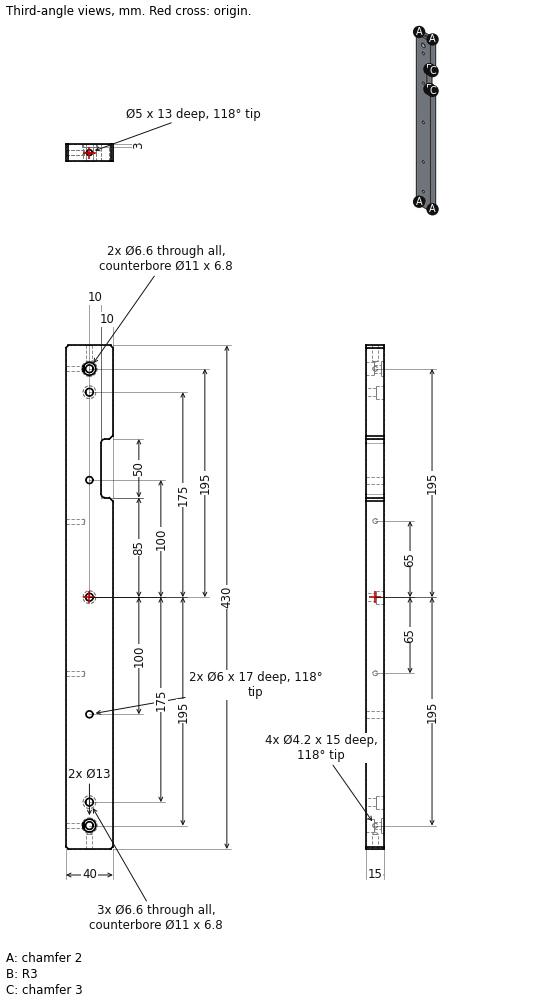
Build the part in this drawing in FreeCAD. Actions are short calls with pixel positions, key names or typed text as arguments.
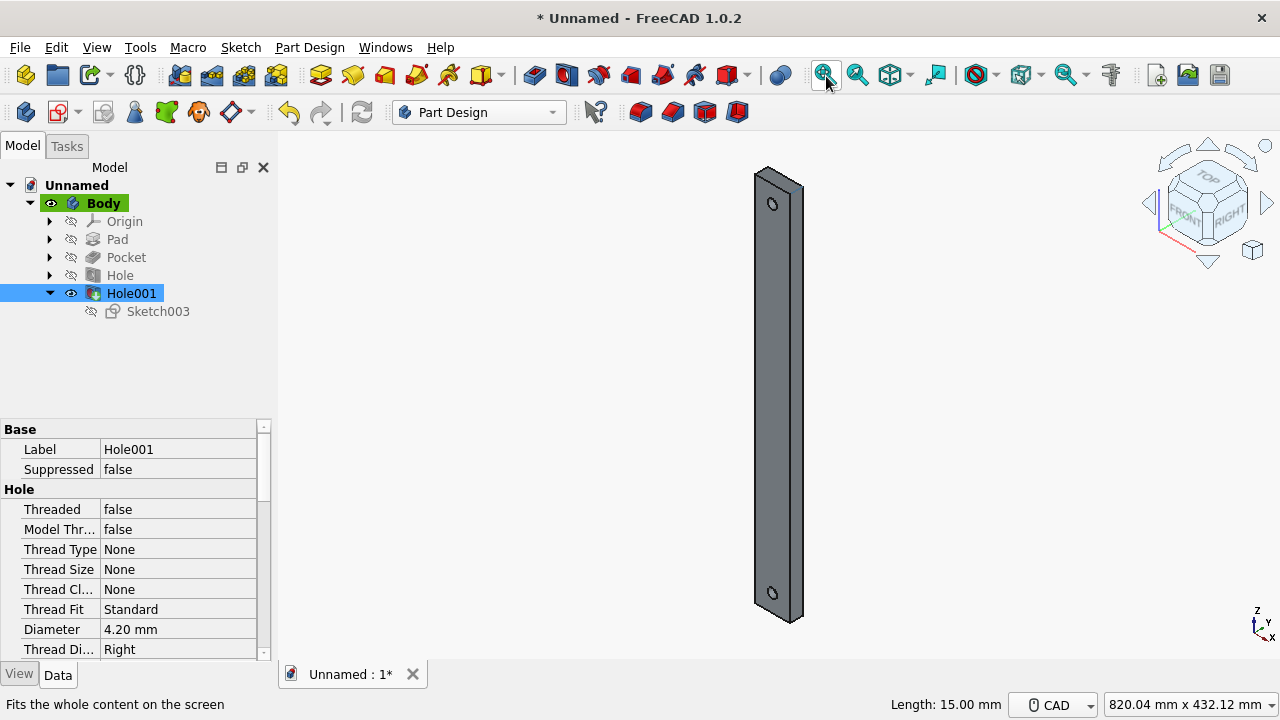
key(2)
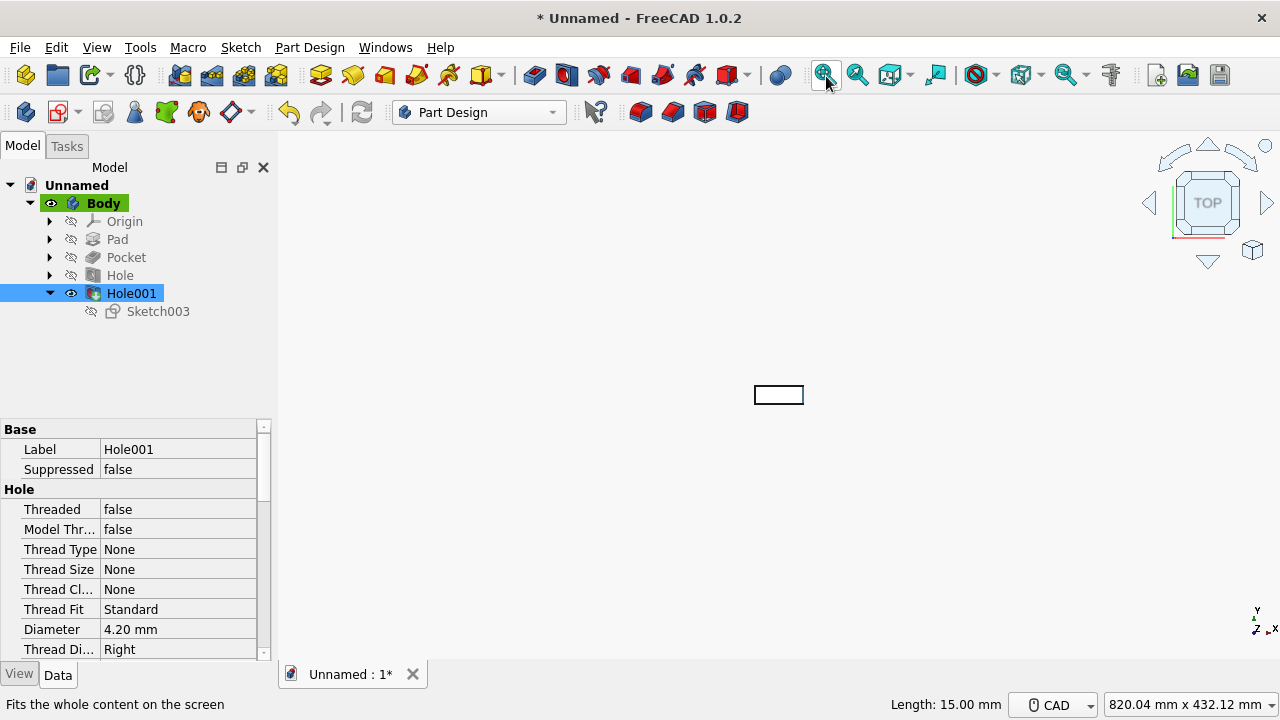
click(826, 76)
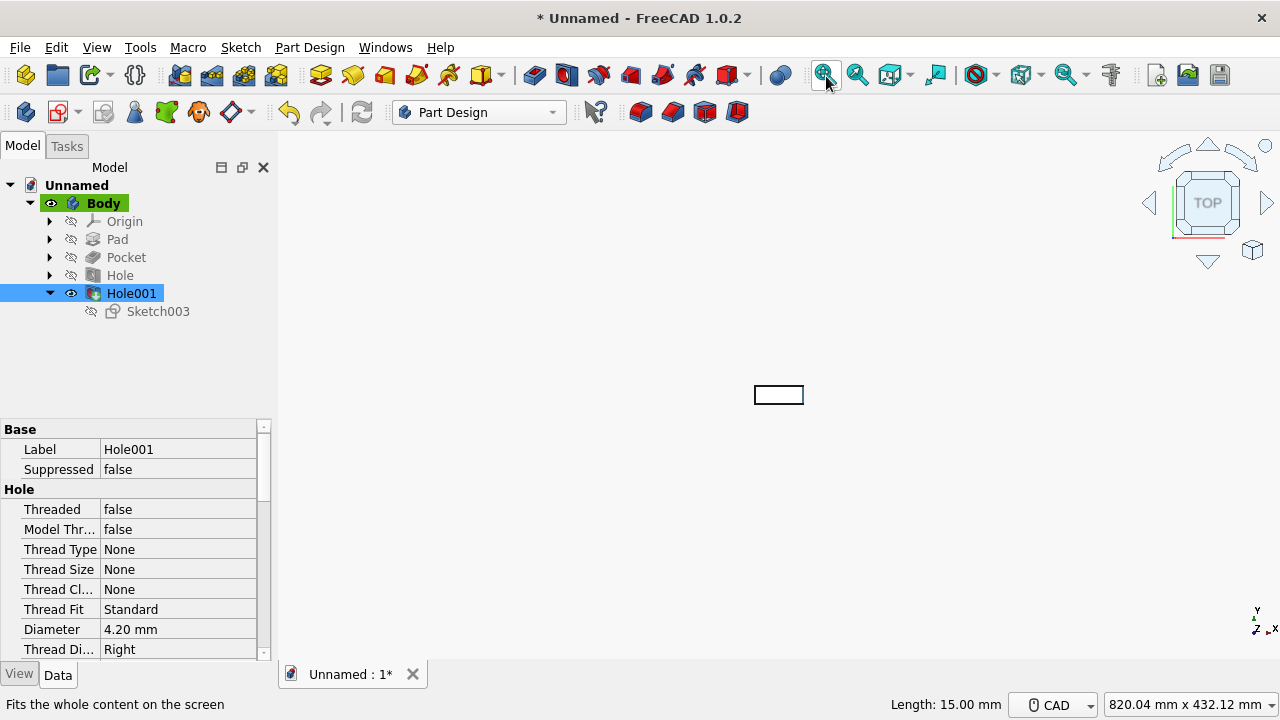
click(755, 394, ctrl)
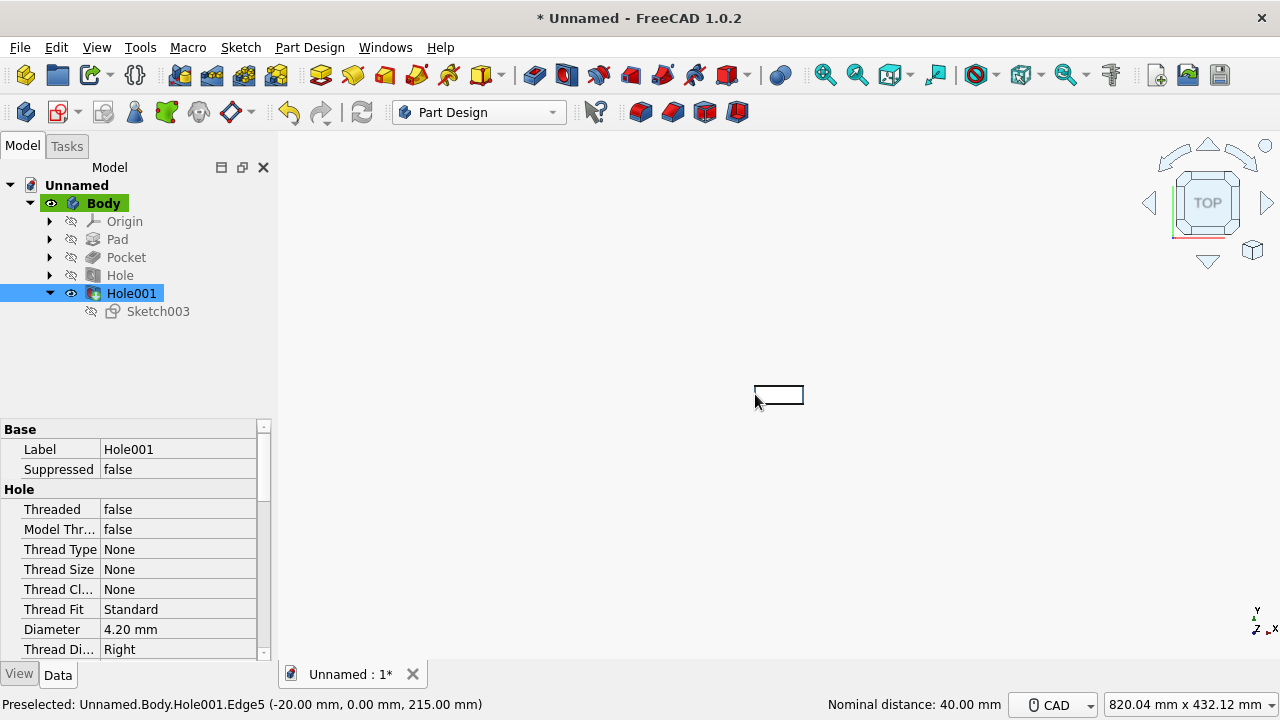
scroll(755, 394, up, 4)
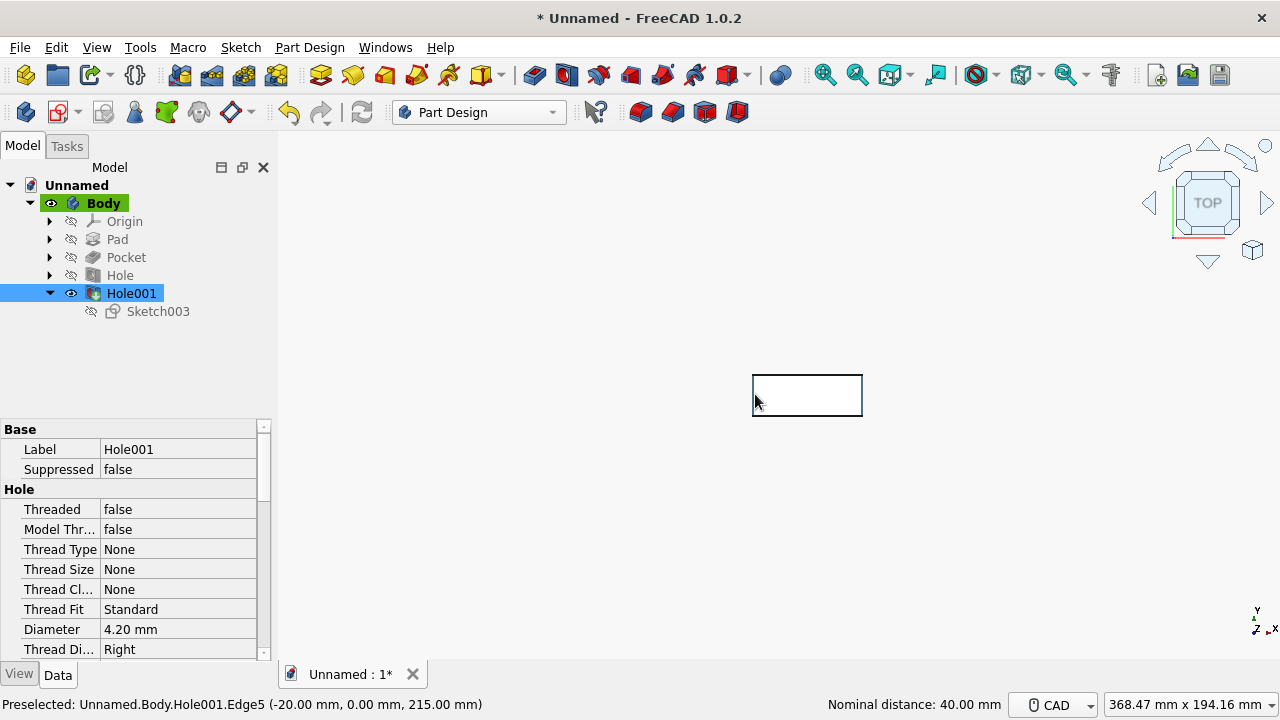
click(826, 76)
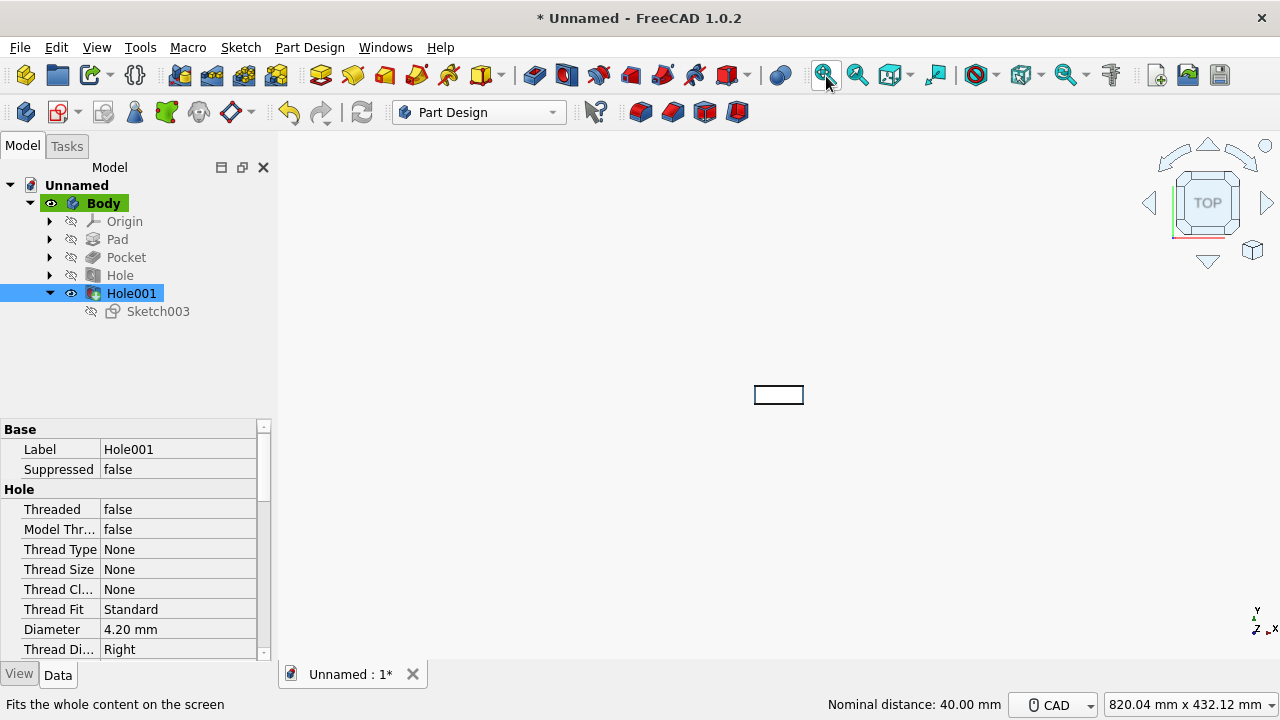
key(1)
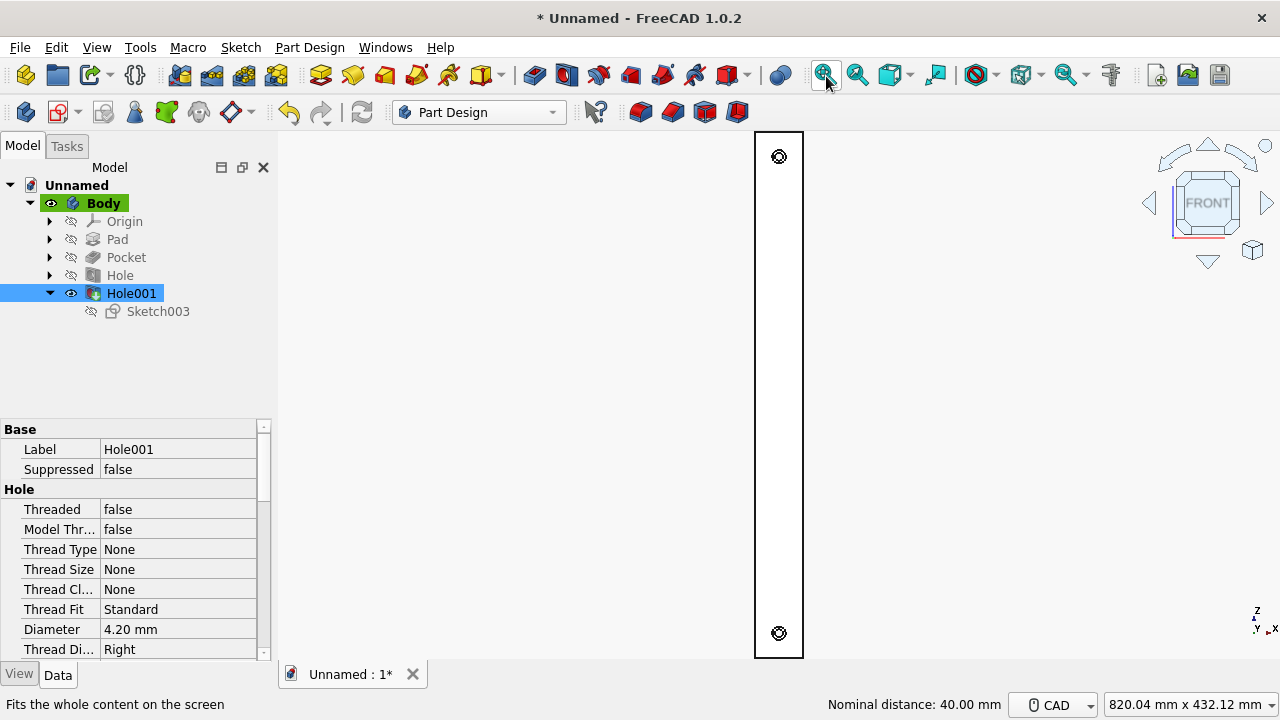
key(3)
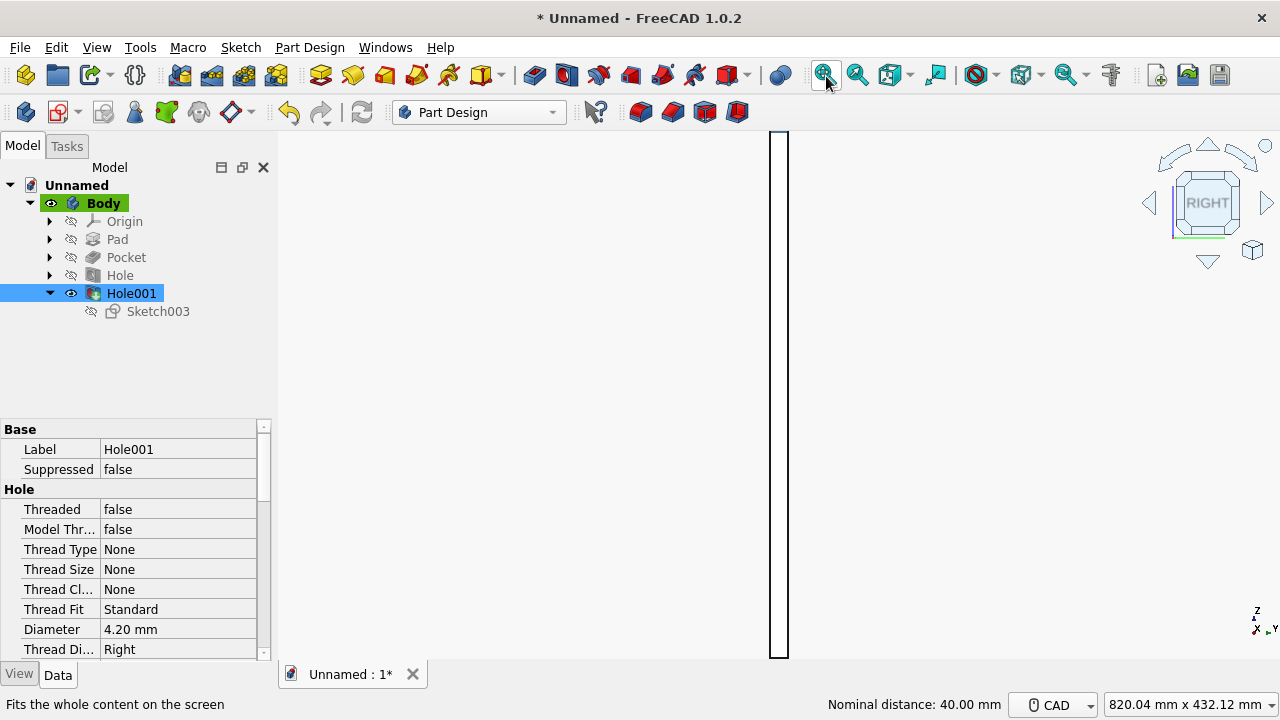
key(5)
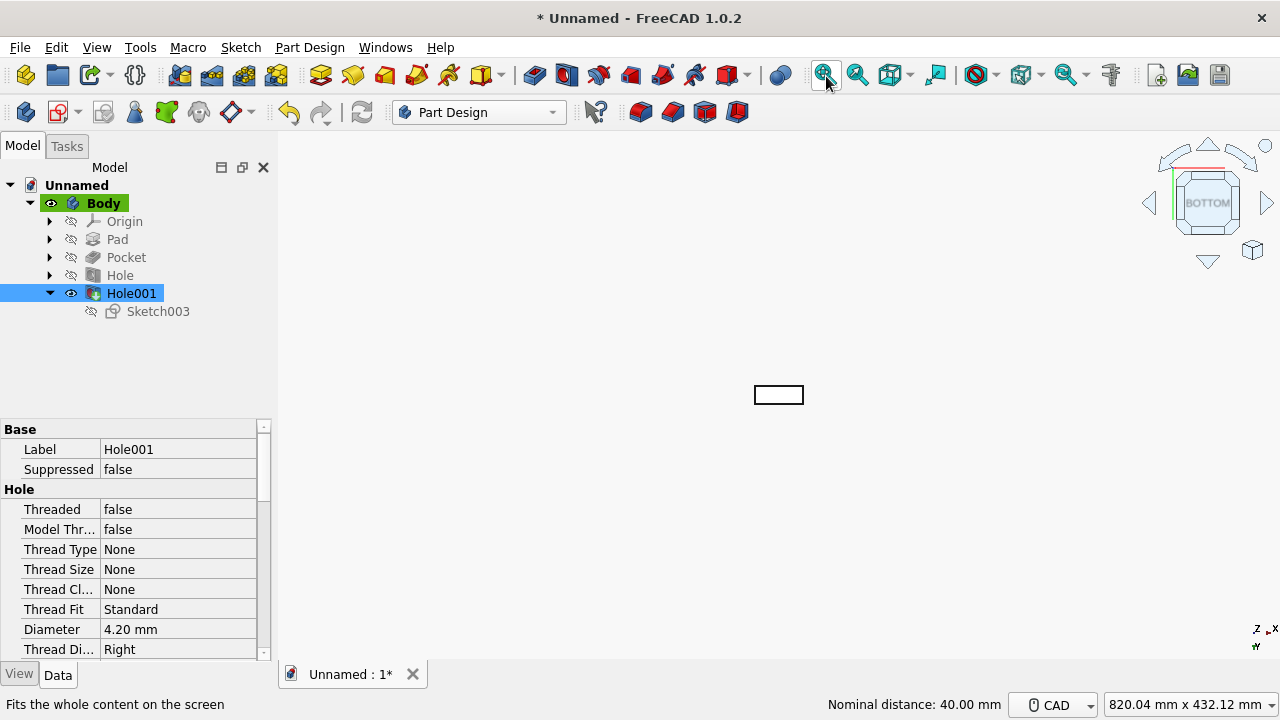
click(826, 76)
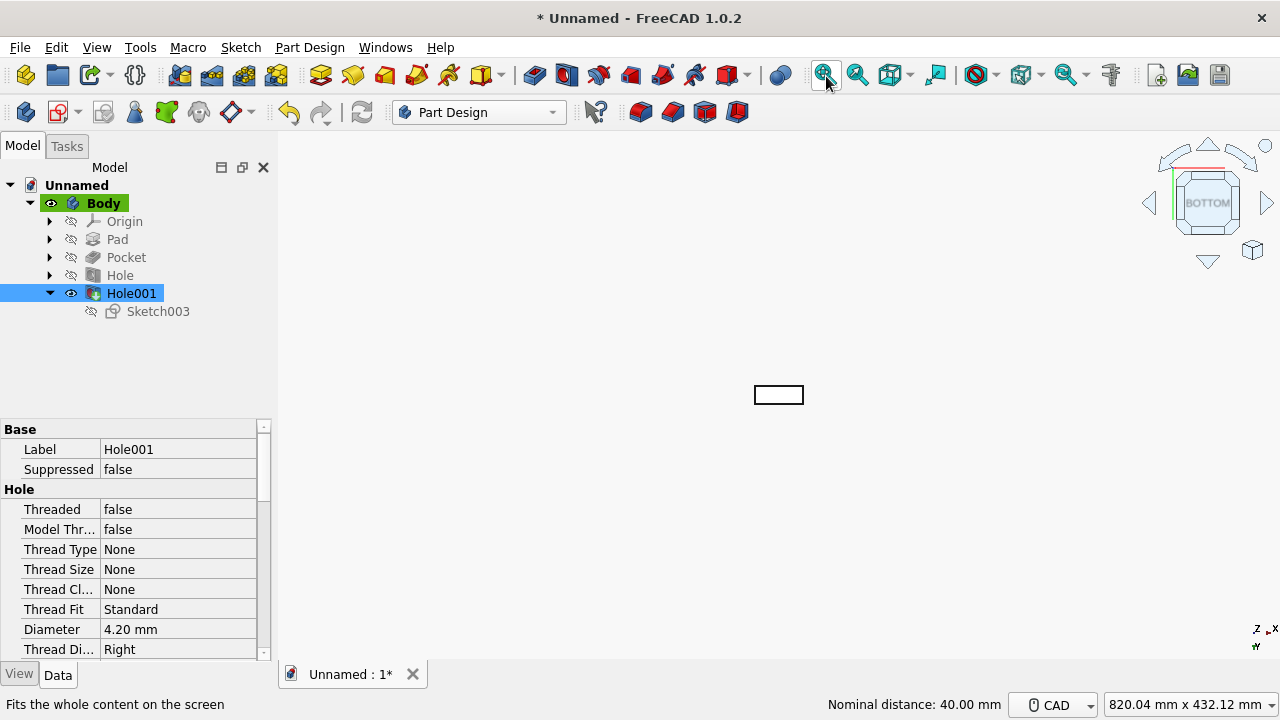
click(755, 394, ctrl)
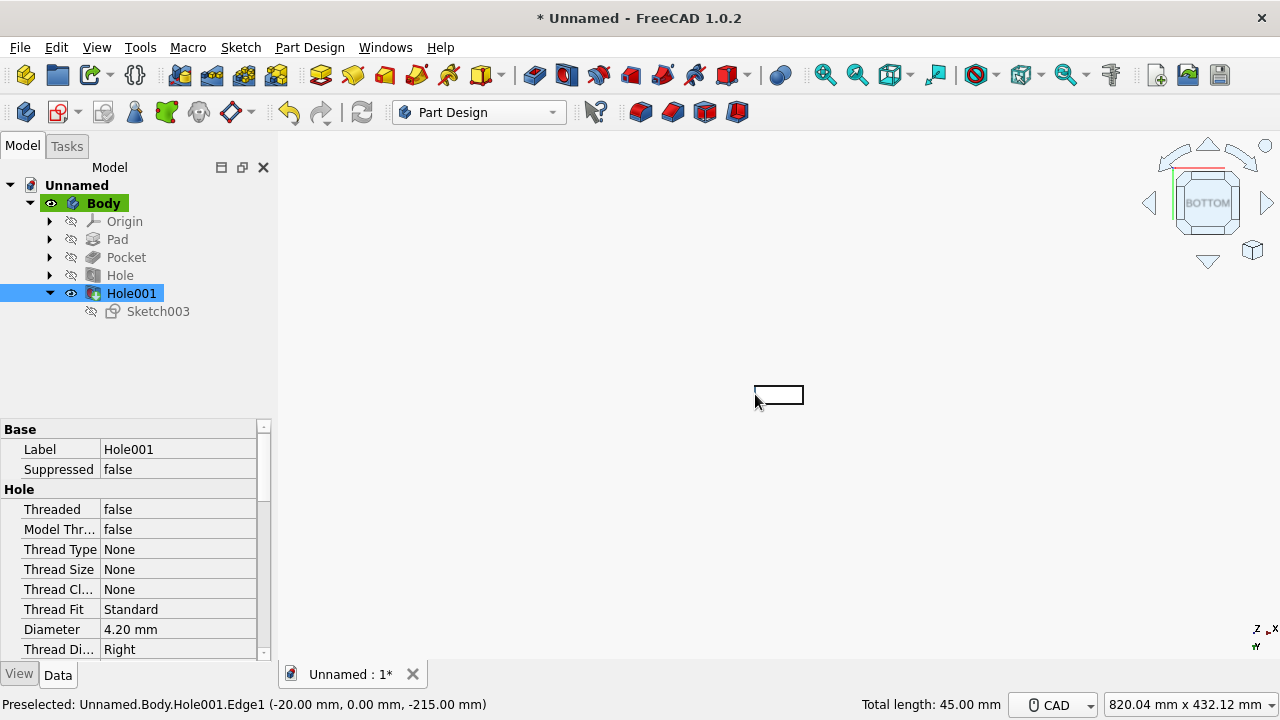
click(803, 394, ctrl)